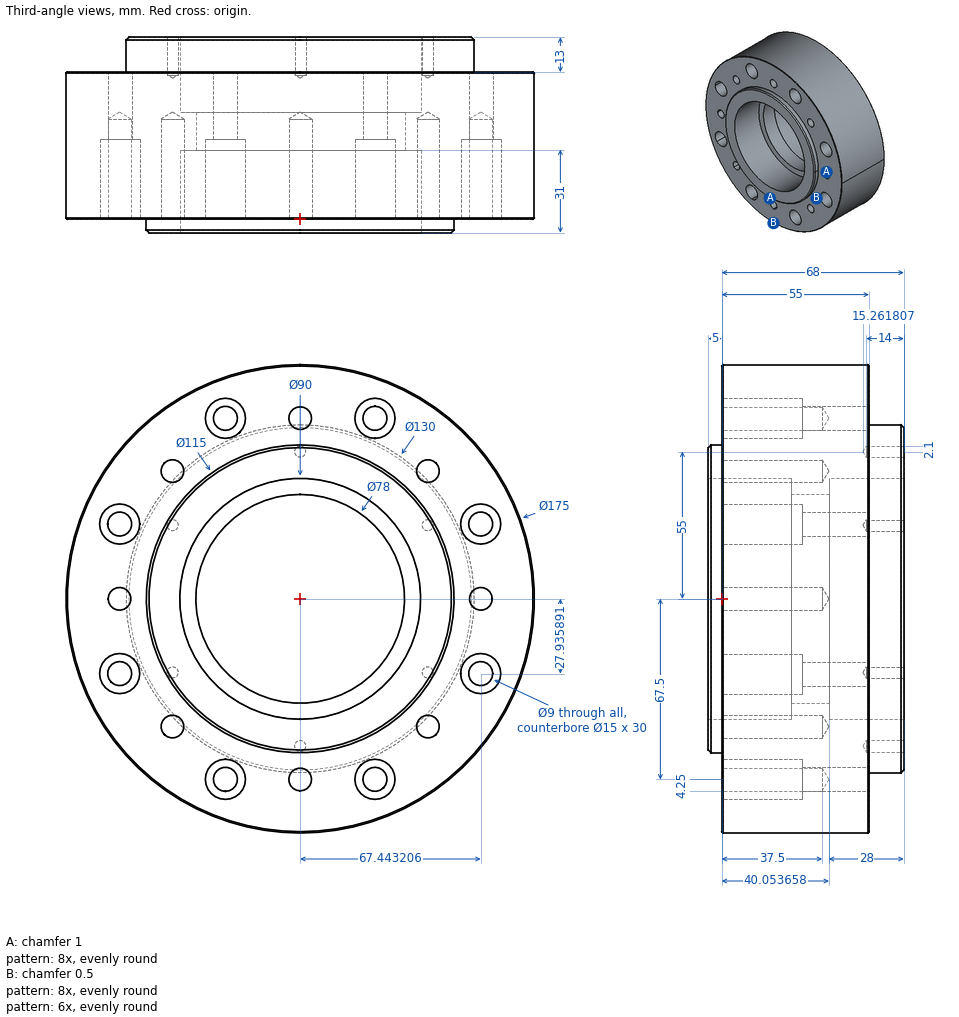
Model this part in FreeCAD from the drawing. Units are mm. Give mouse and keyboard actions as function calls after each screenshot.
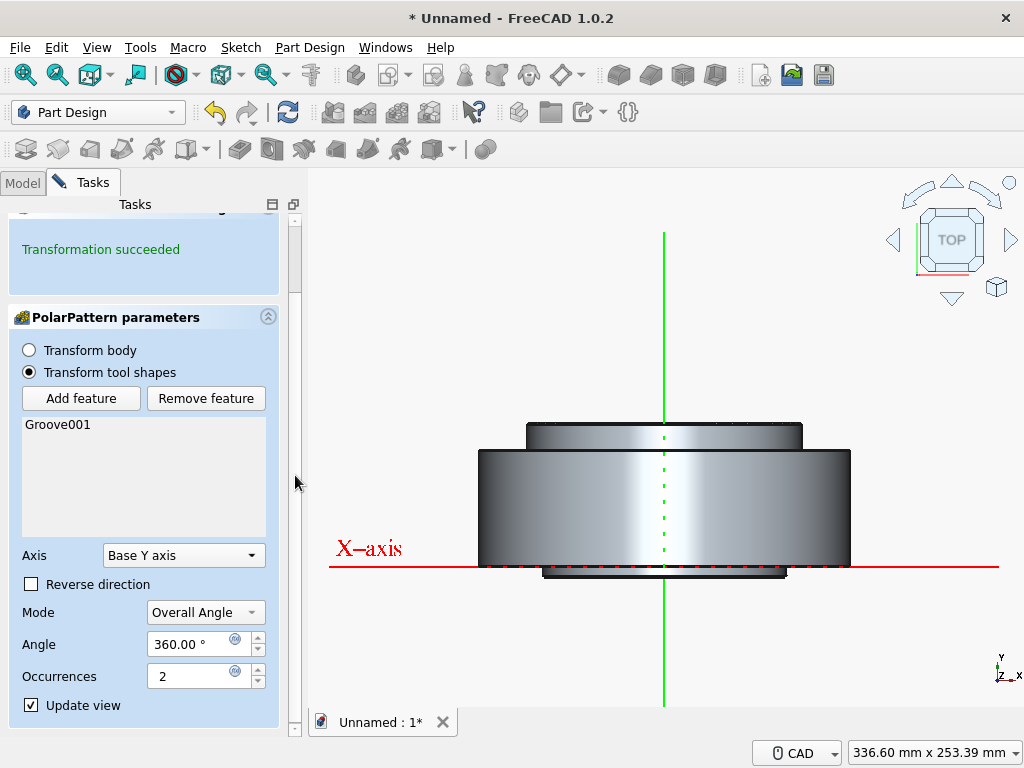
triple_click(198, 676)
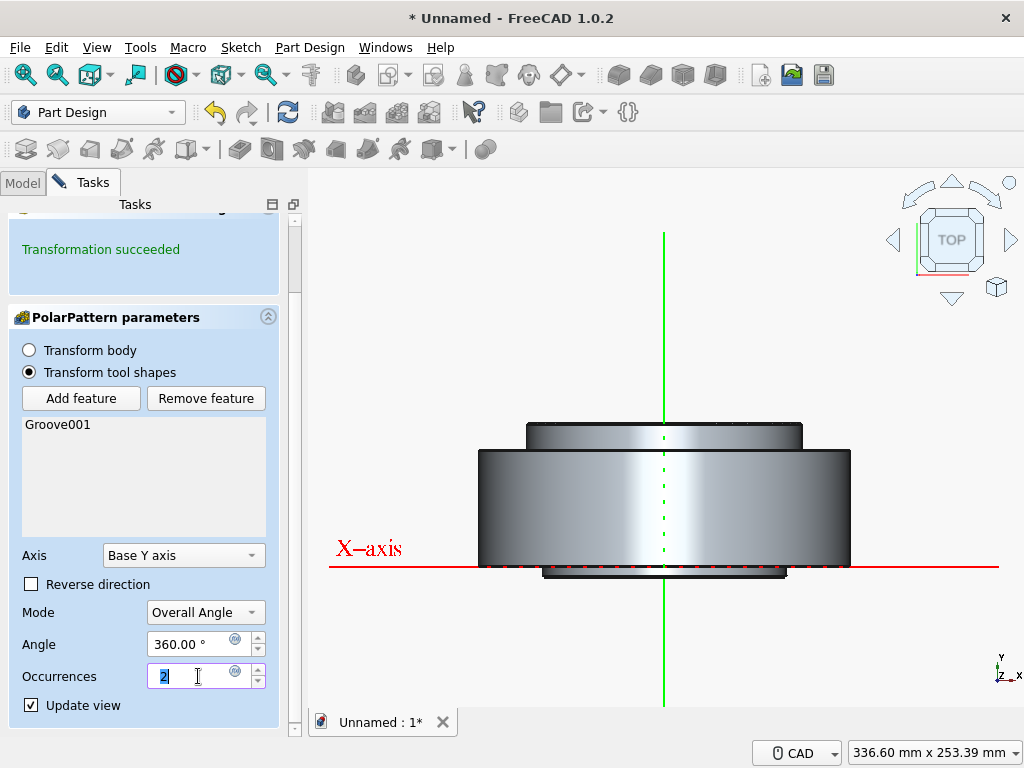
text(6)
key(Tab)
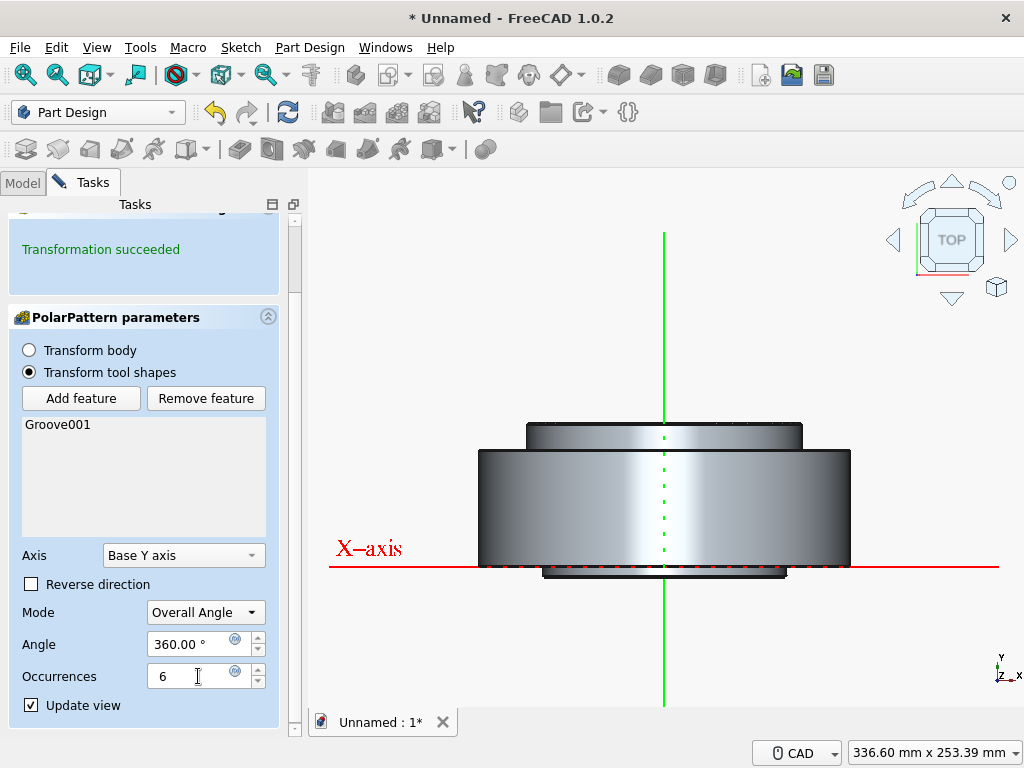
scroll(295, 475, up, 3)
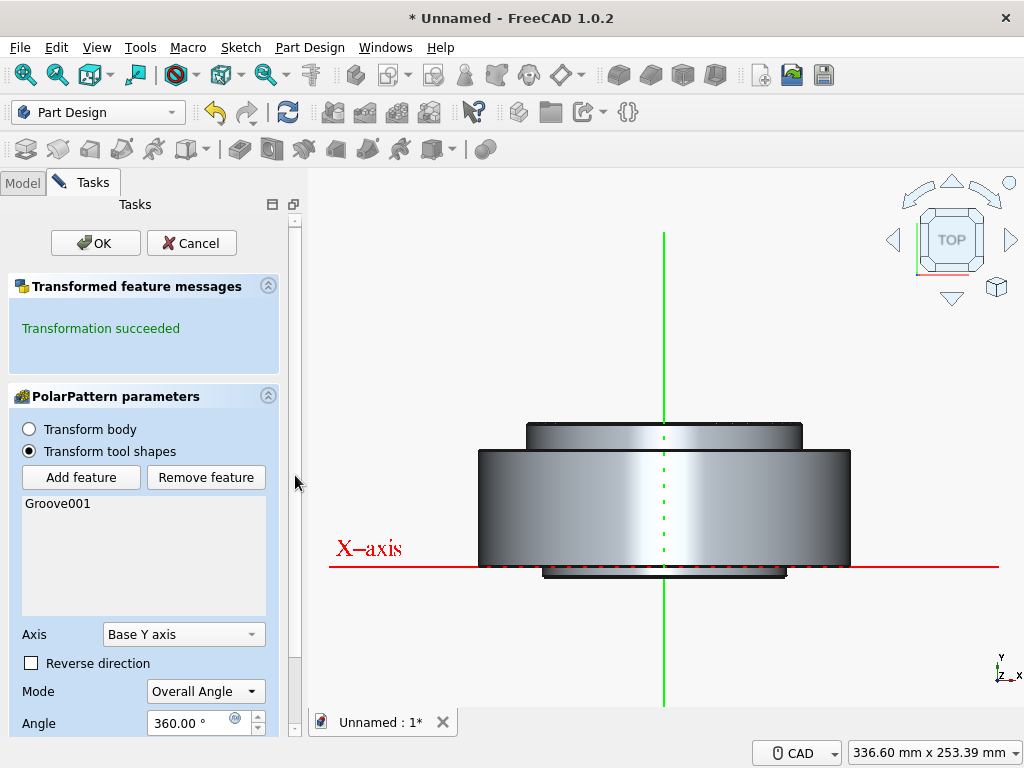
click(96, 243)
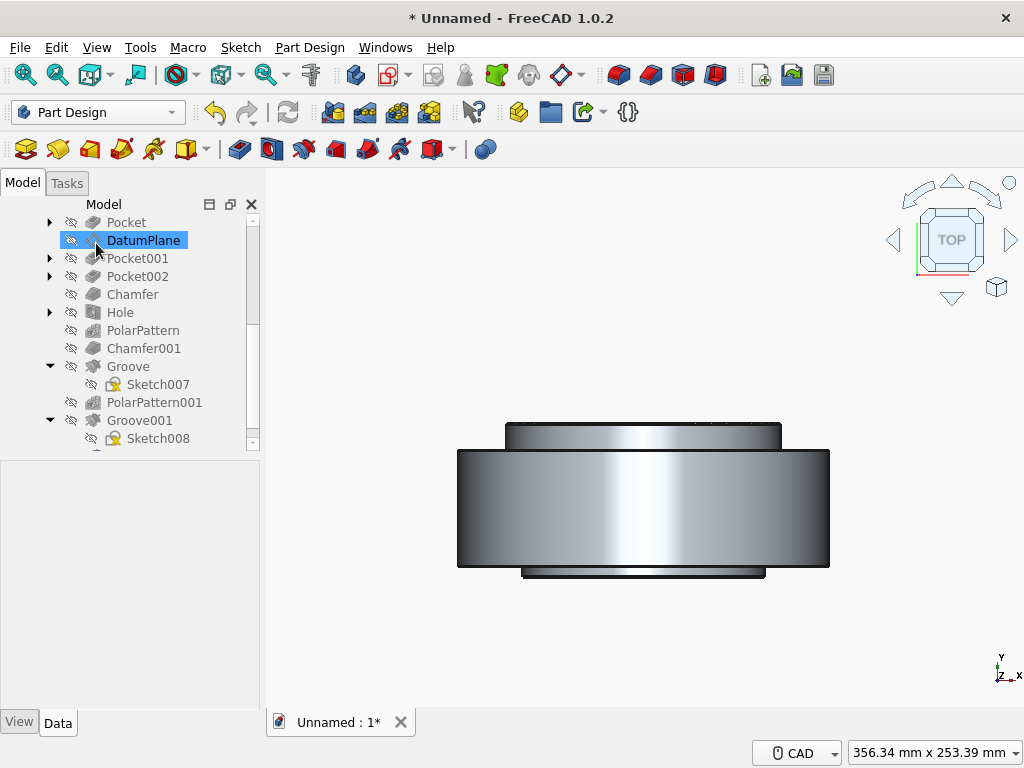
key(0)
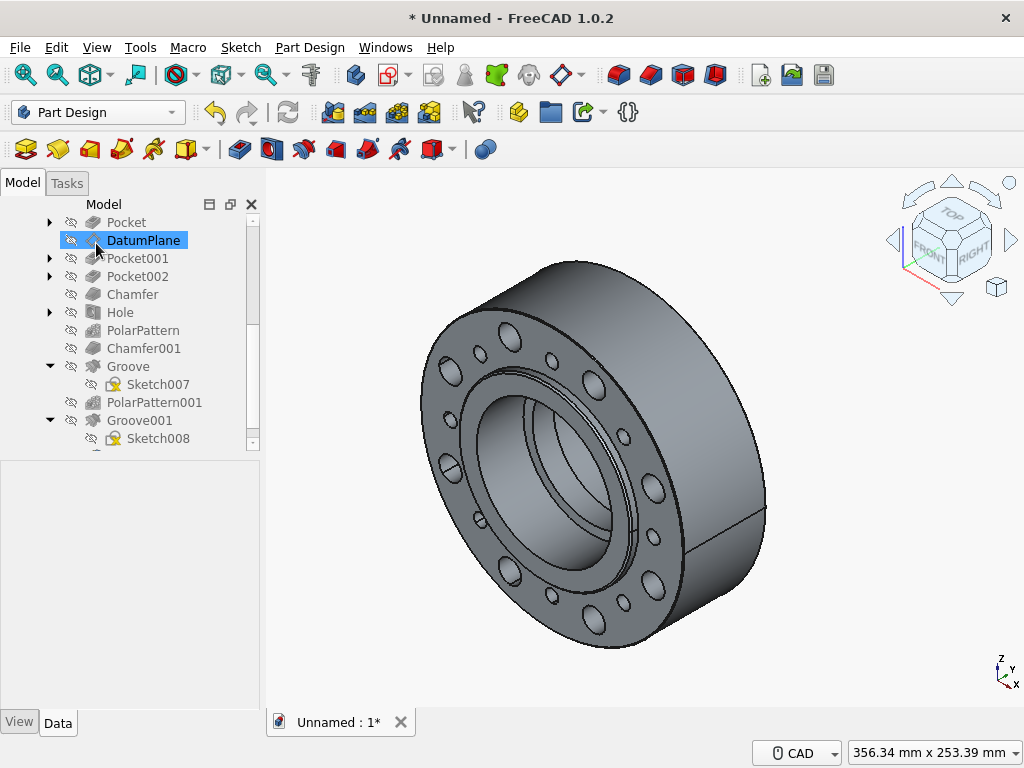
click(26, 76)